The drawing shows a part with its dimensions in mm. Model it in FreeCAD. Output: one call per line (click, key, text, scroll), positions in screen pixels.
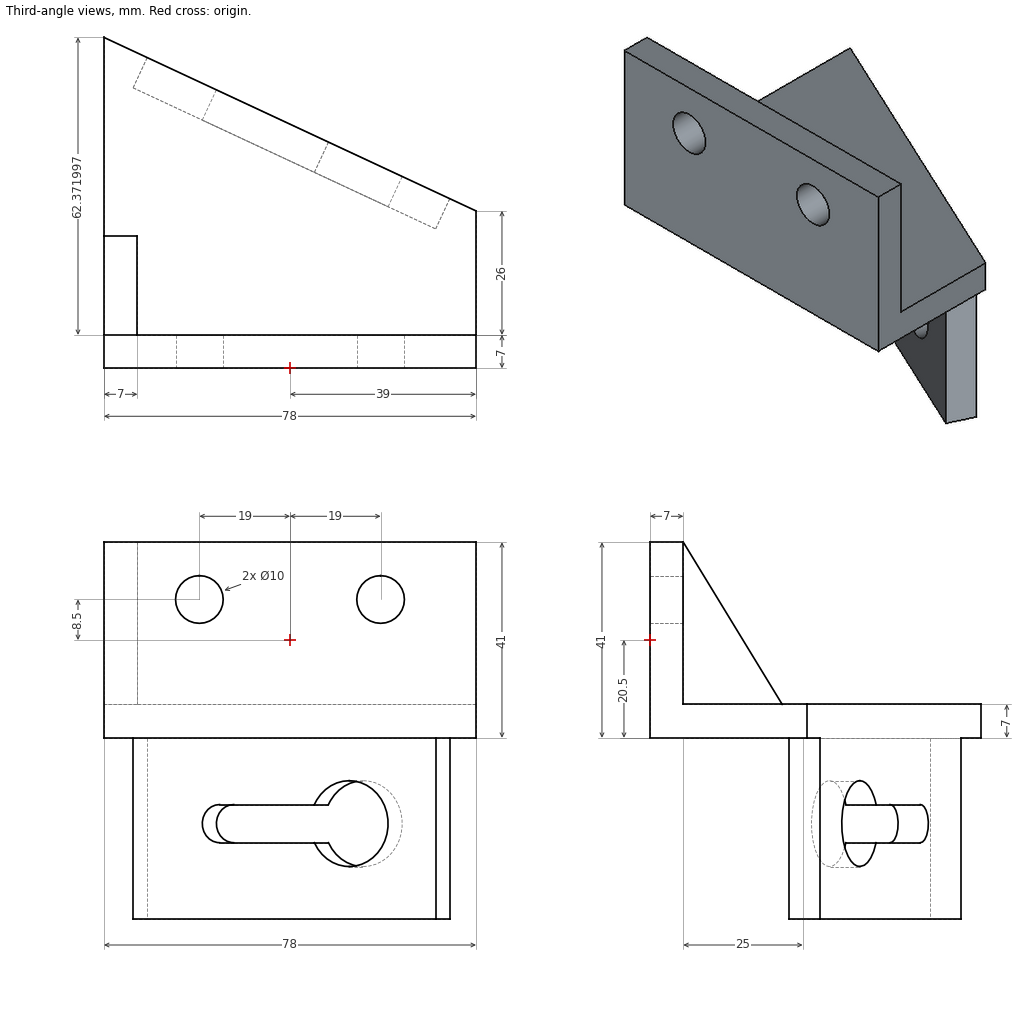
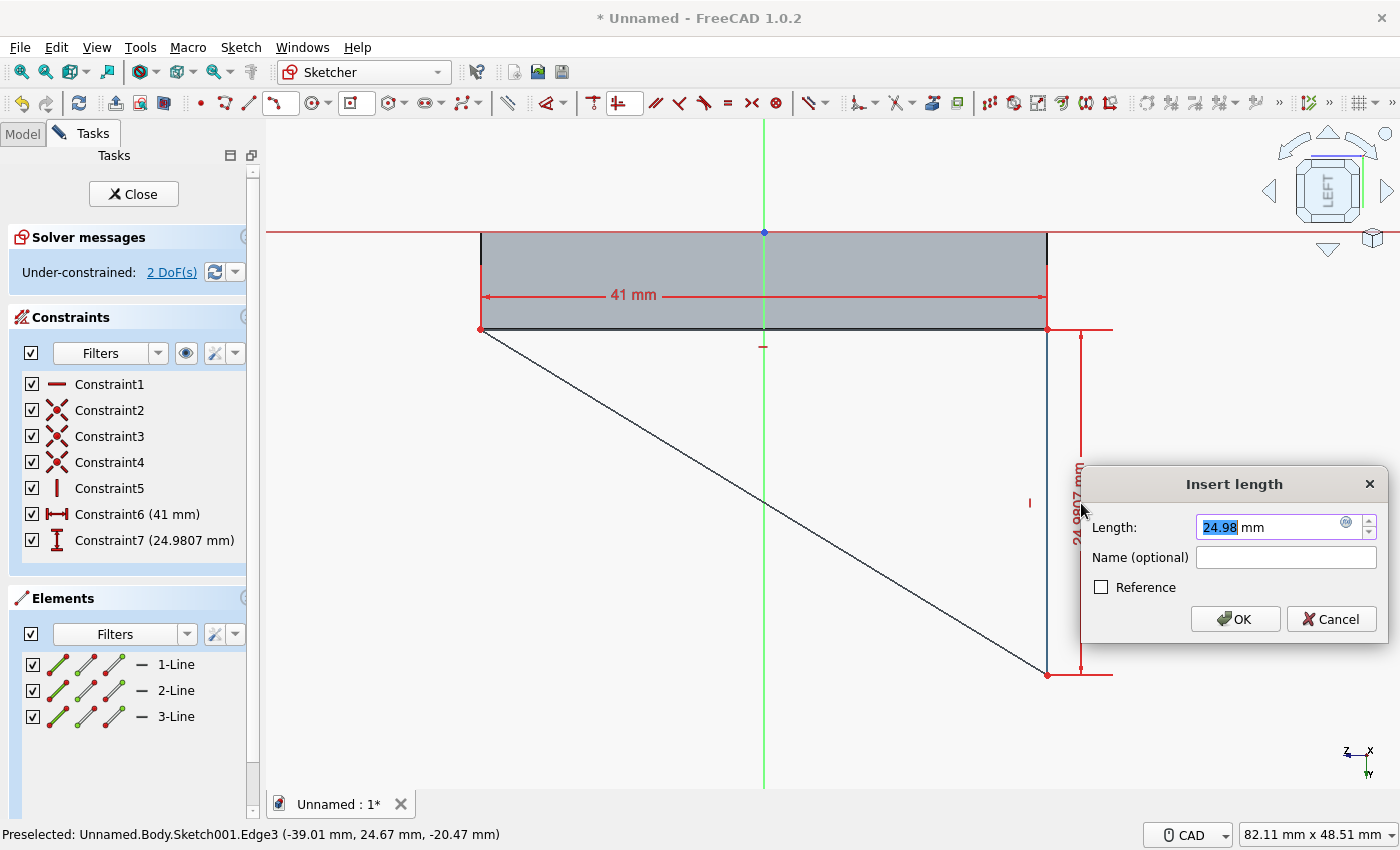
text(25)
key(Return)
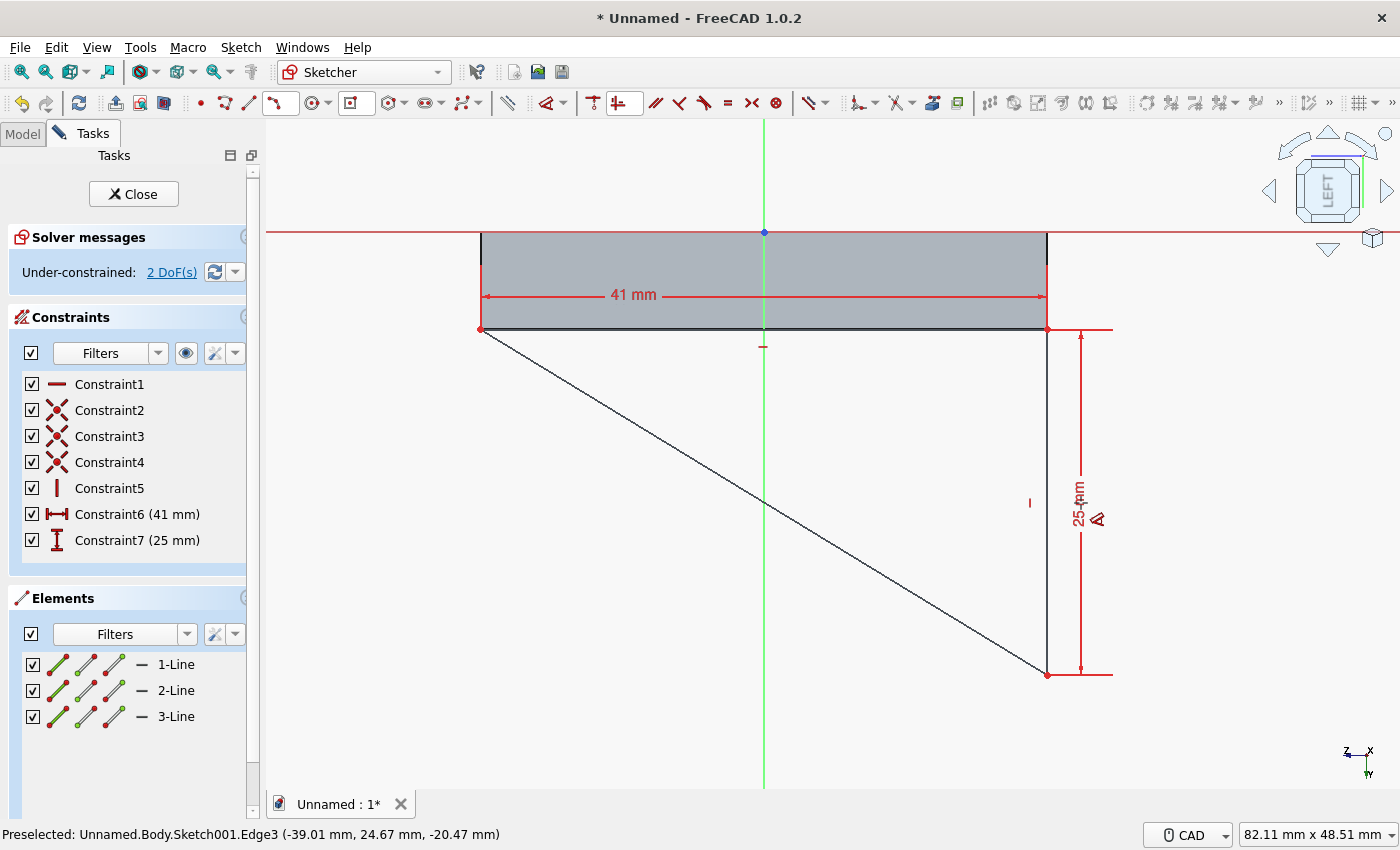
click(1047, 330)
click(1081, 281)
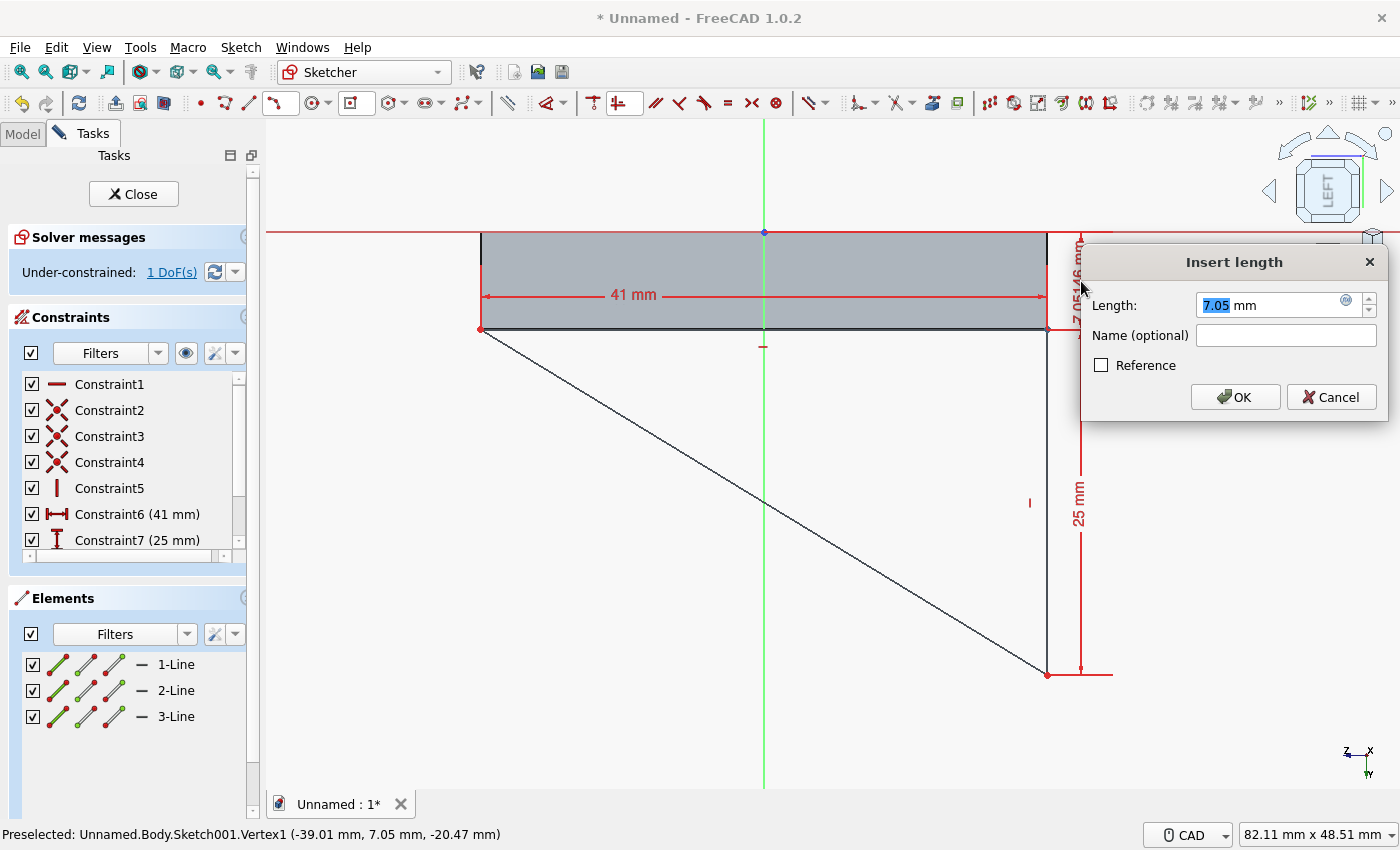
text(7)
key(Return)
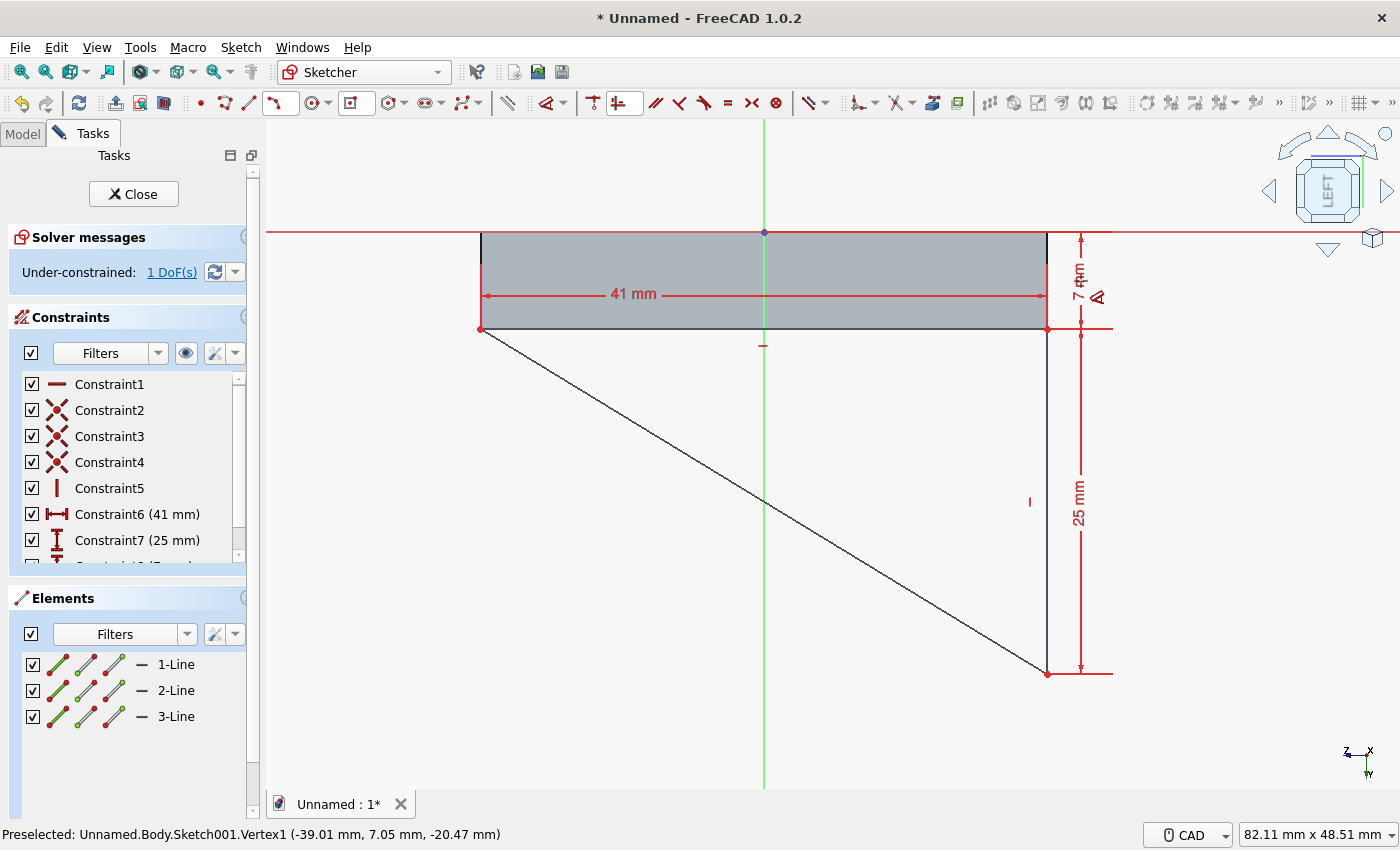
click(1047, 329)
click(906, 198)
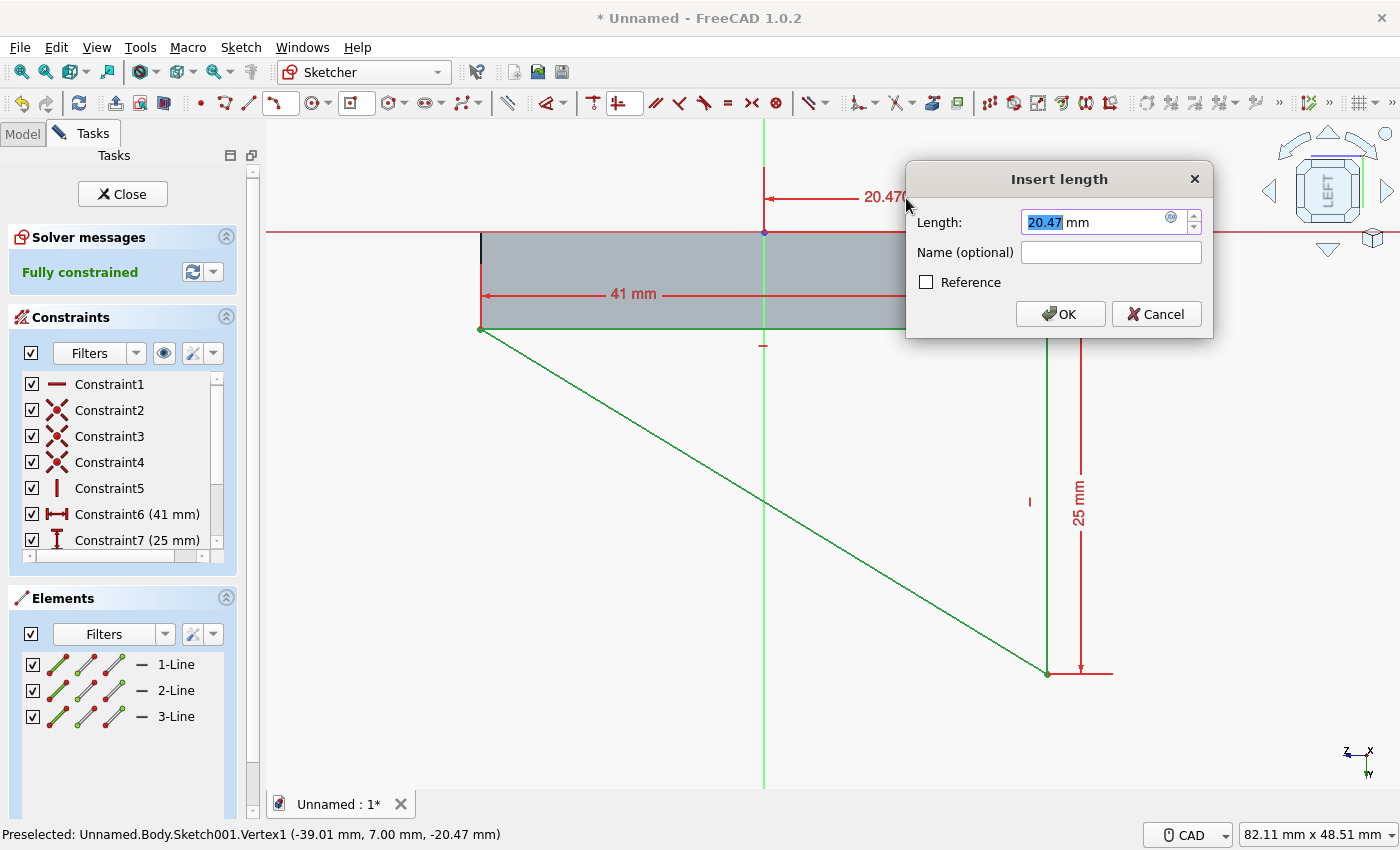
text(20.5)
key(Return)
key(Escape)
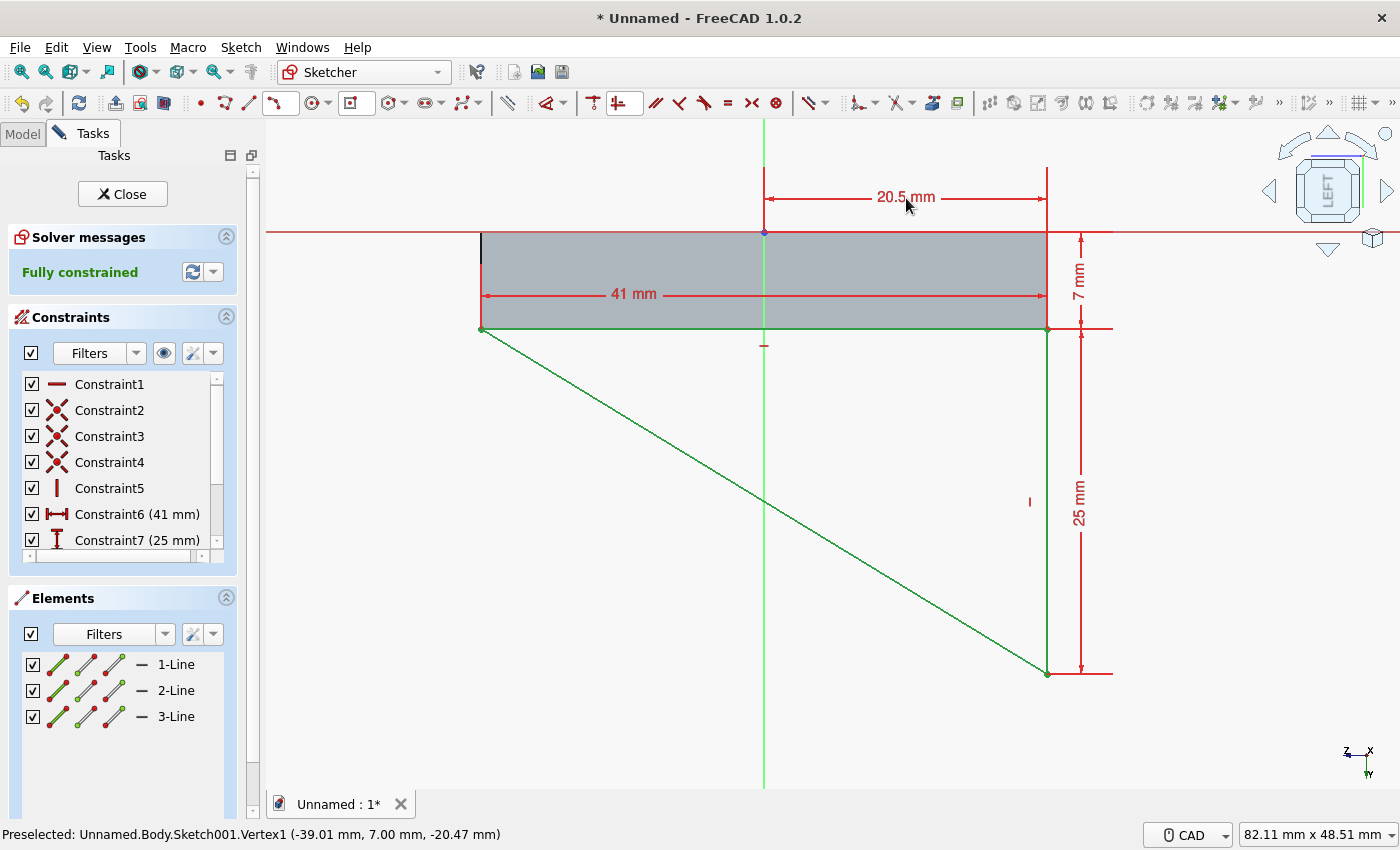
click(123, 194)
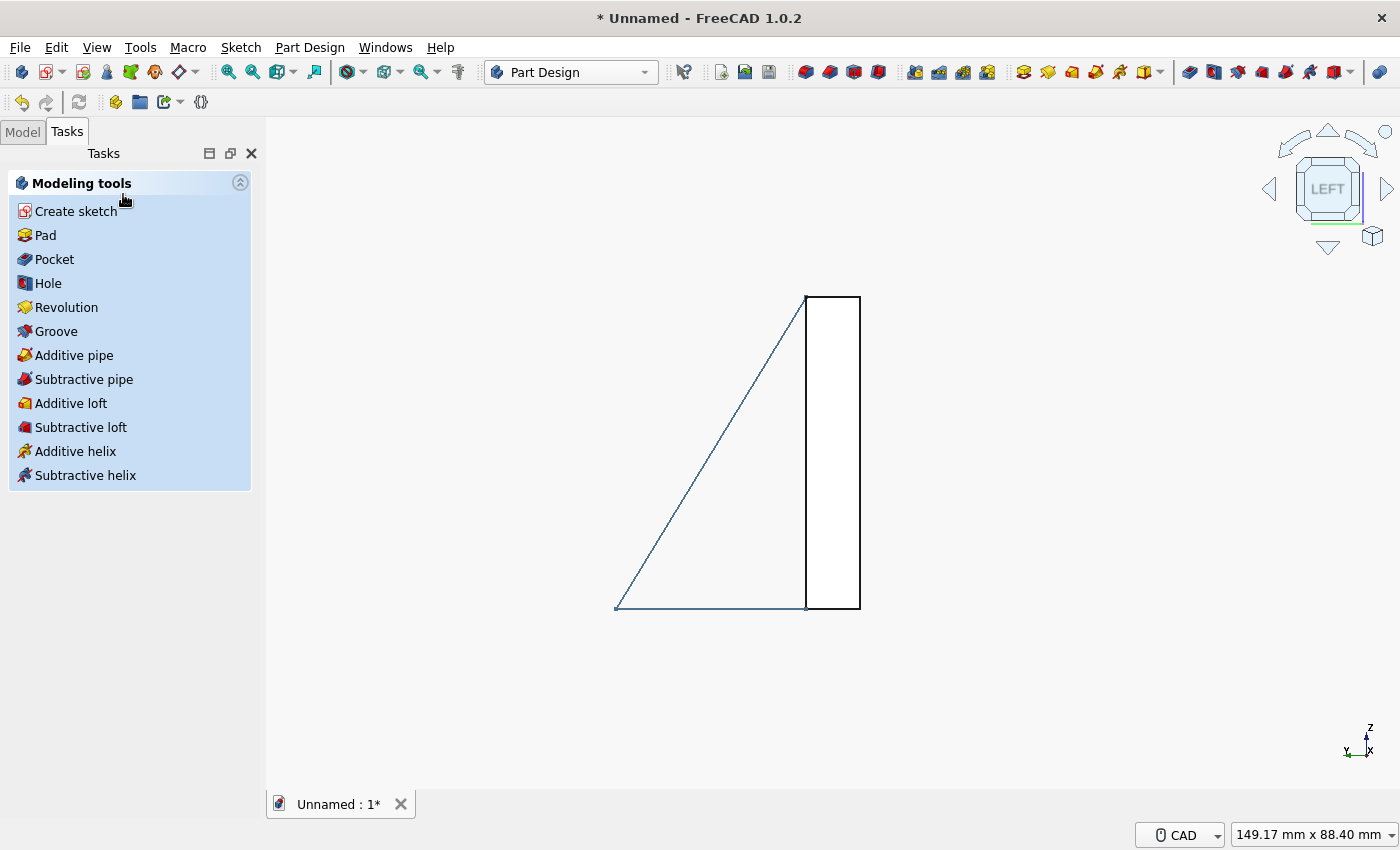
click(1024, 72)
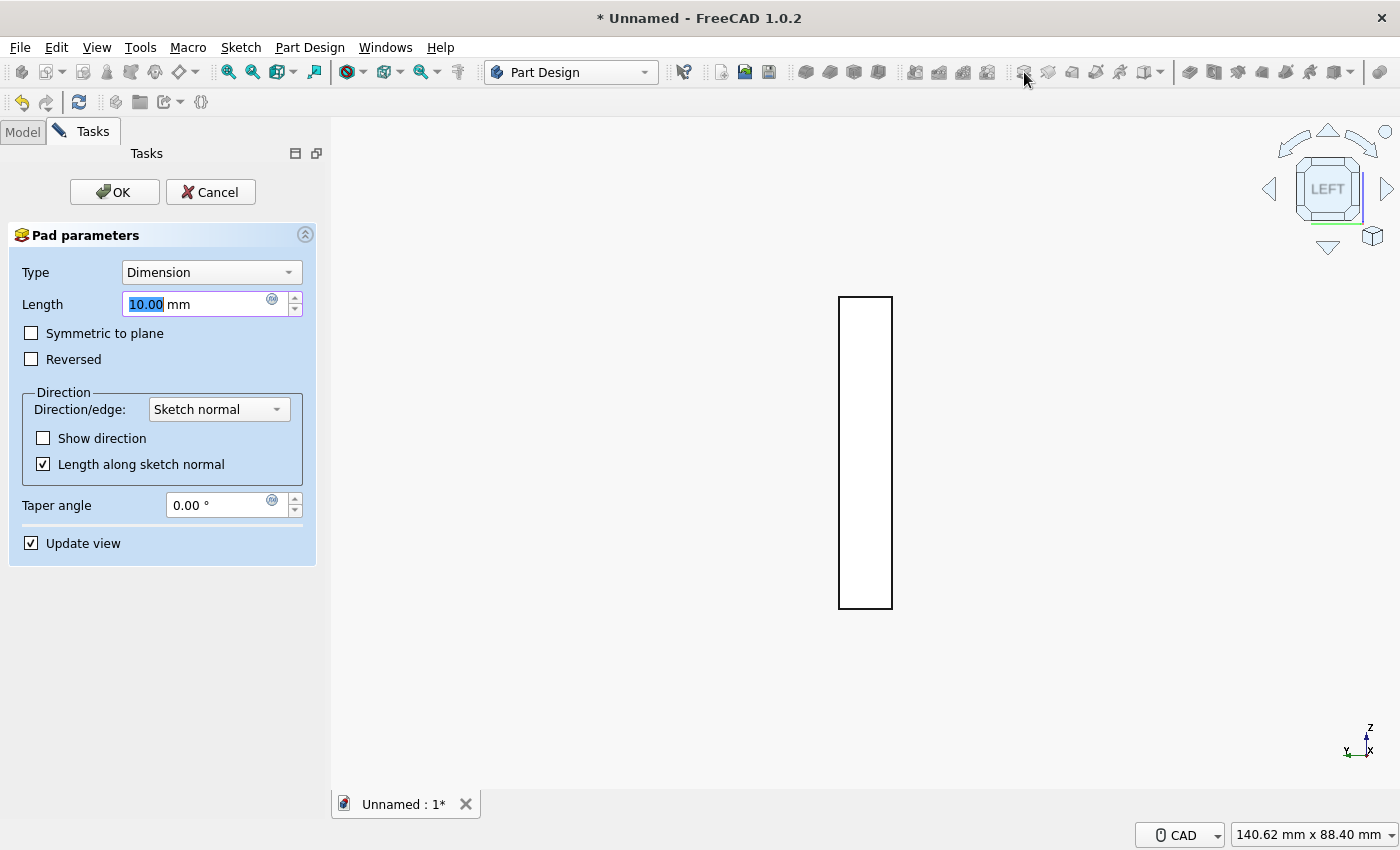
text(7)
key(Tab)